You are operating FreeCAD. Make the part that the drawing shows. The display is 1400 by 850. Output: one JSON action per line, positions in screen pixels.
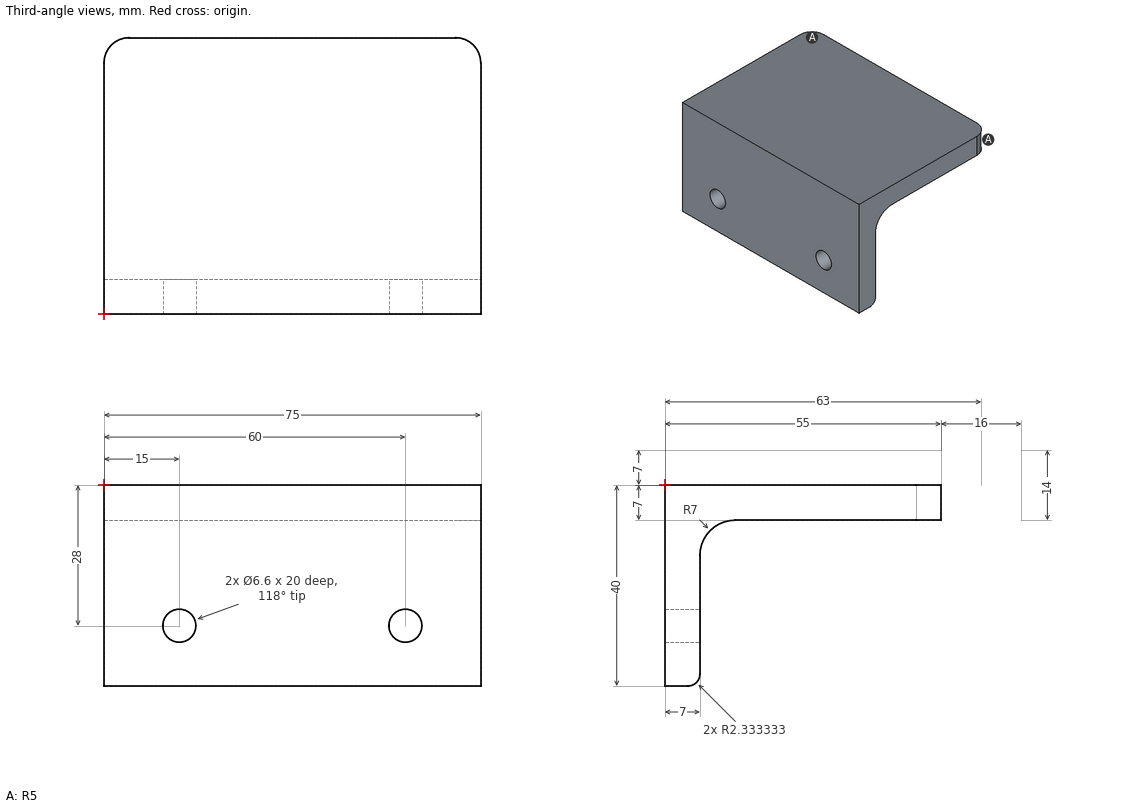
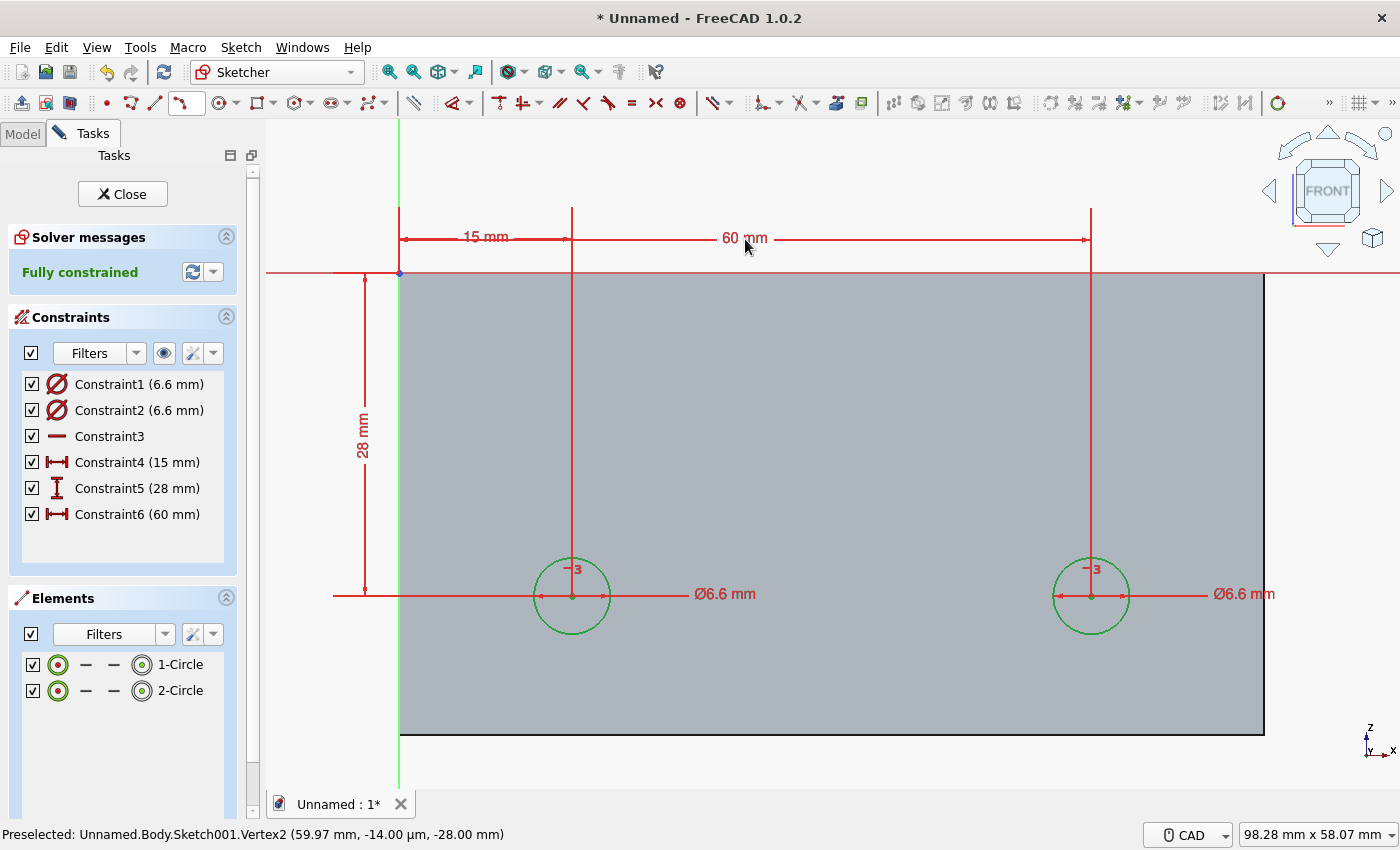
{"action": "left_click", "coordinate": [123, 194]}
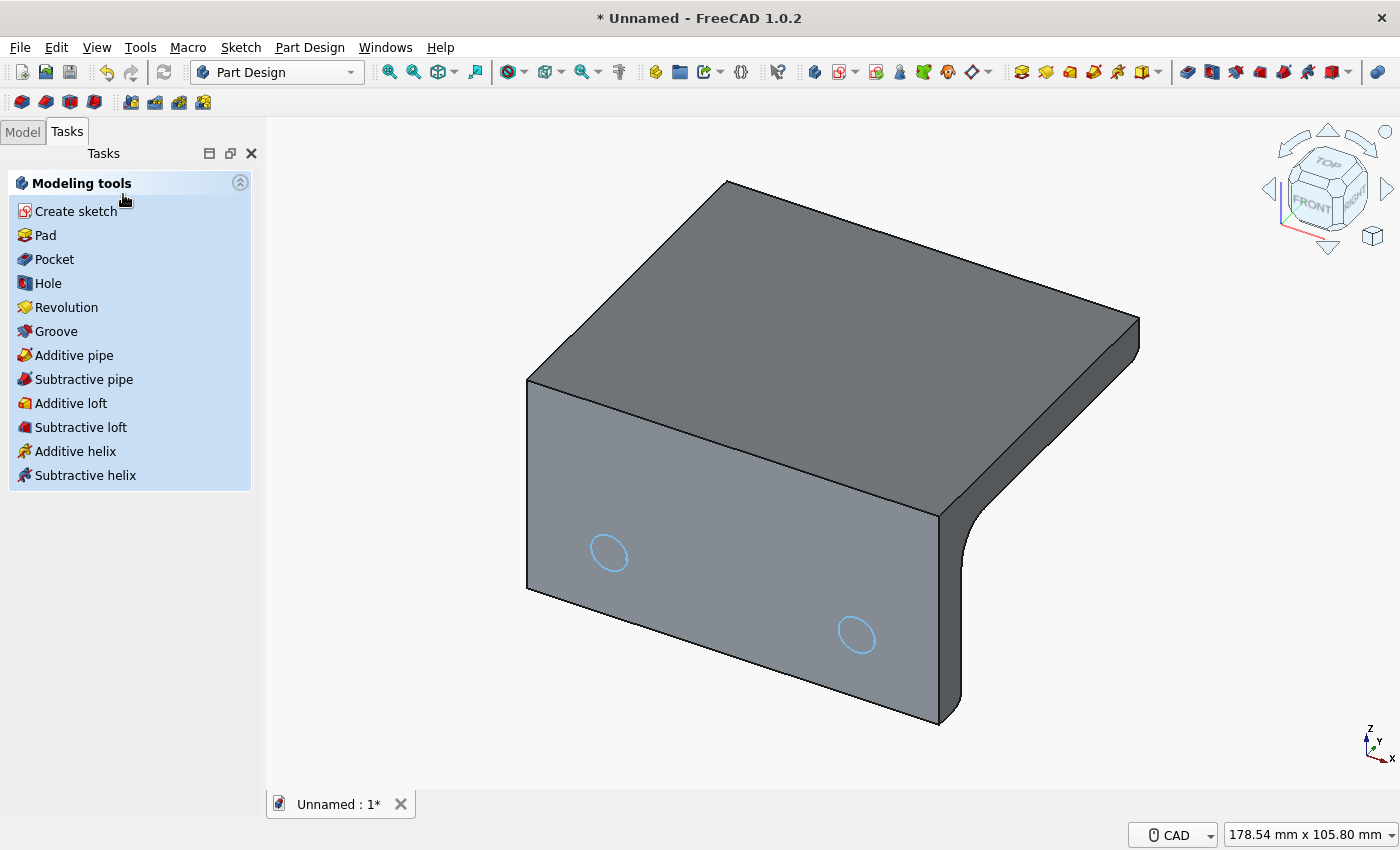
{"action": "left_click", "coordinate": [1212, 72]}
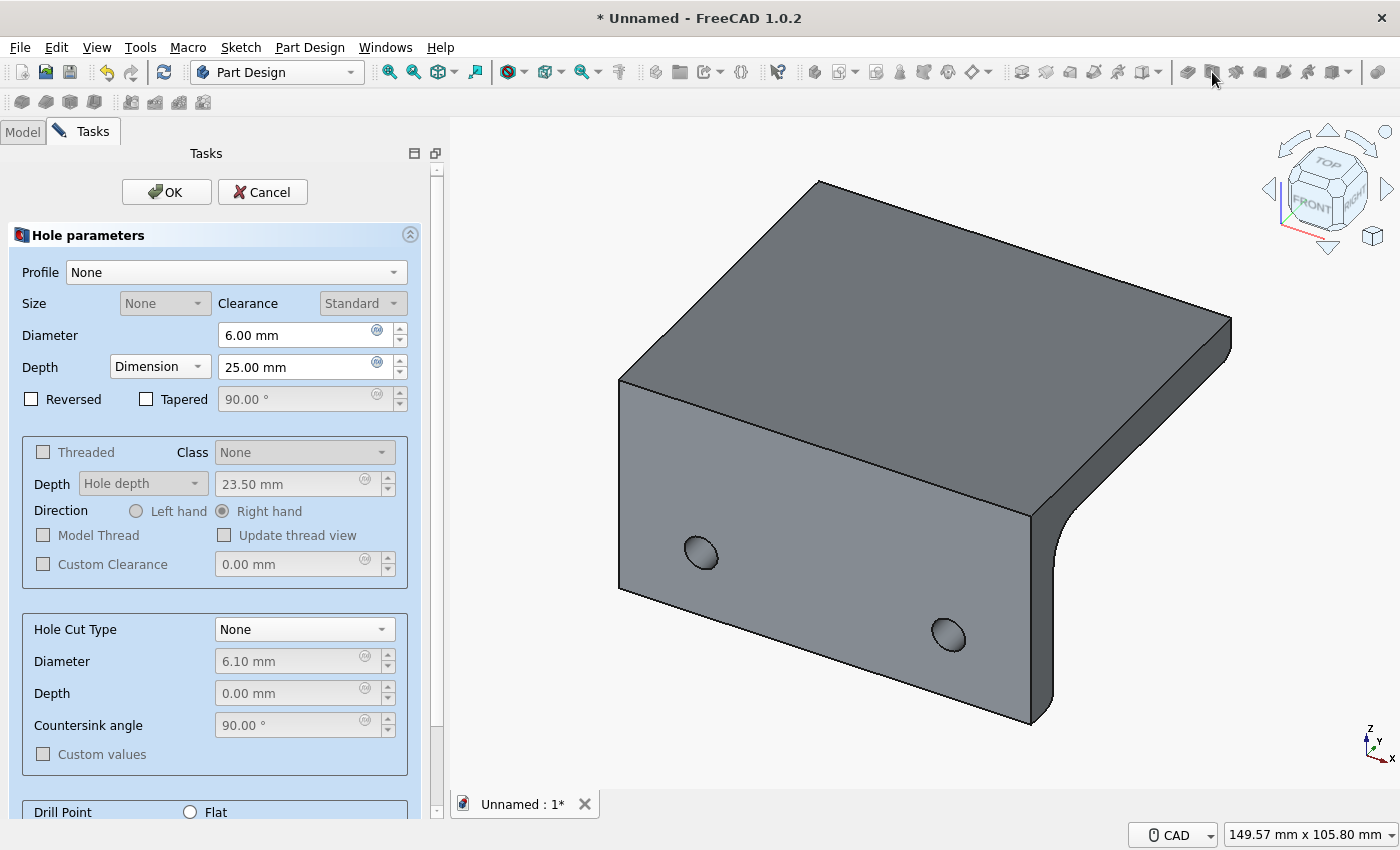
{"action": "triple_click", "coordinate": [305, 335]}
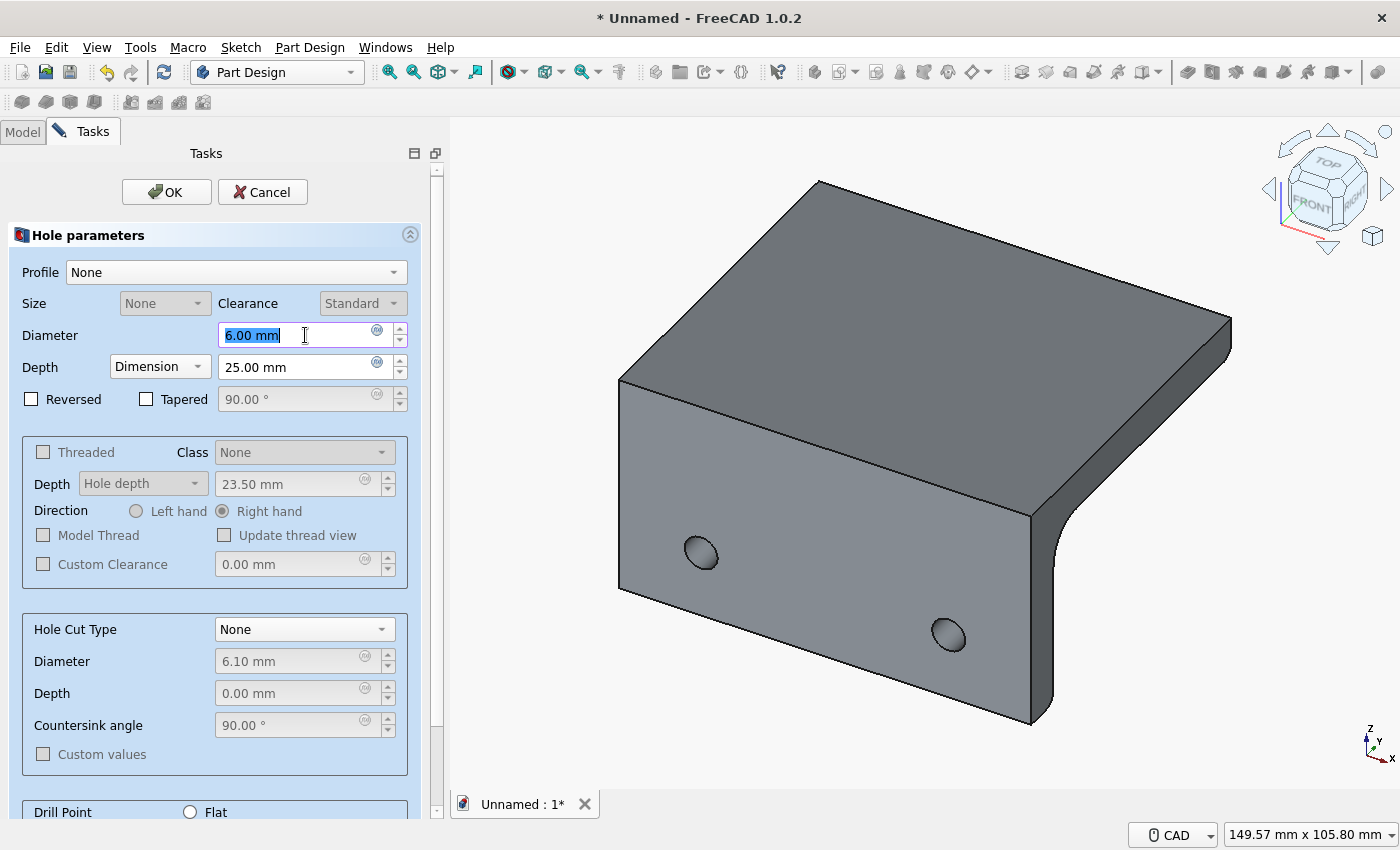
{"action": "type", "text": "6.6"}
{"action": "key", "text": "Tab"}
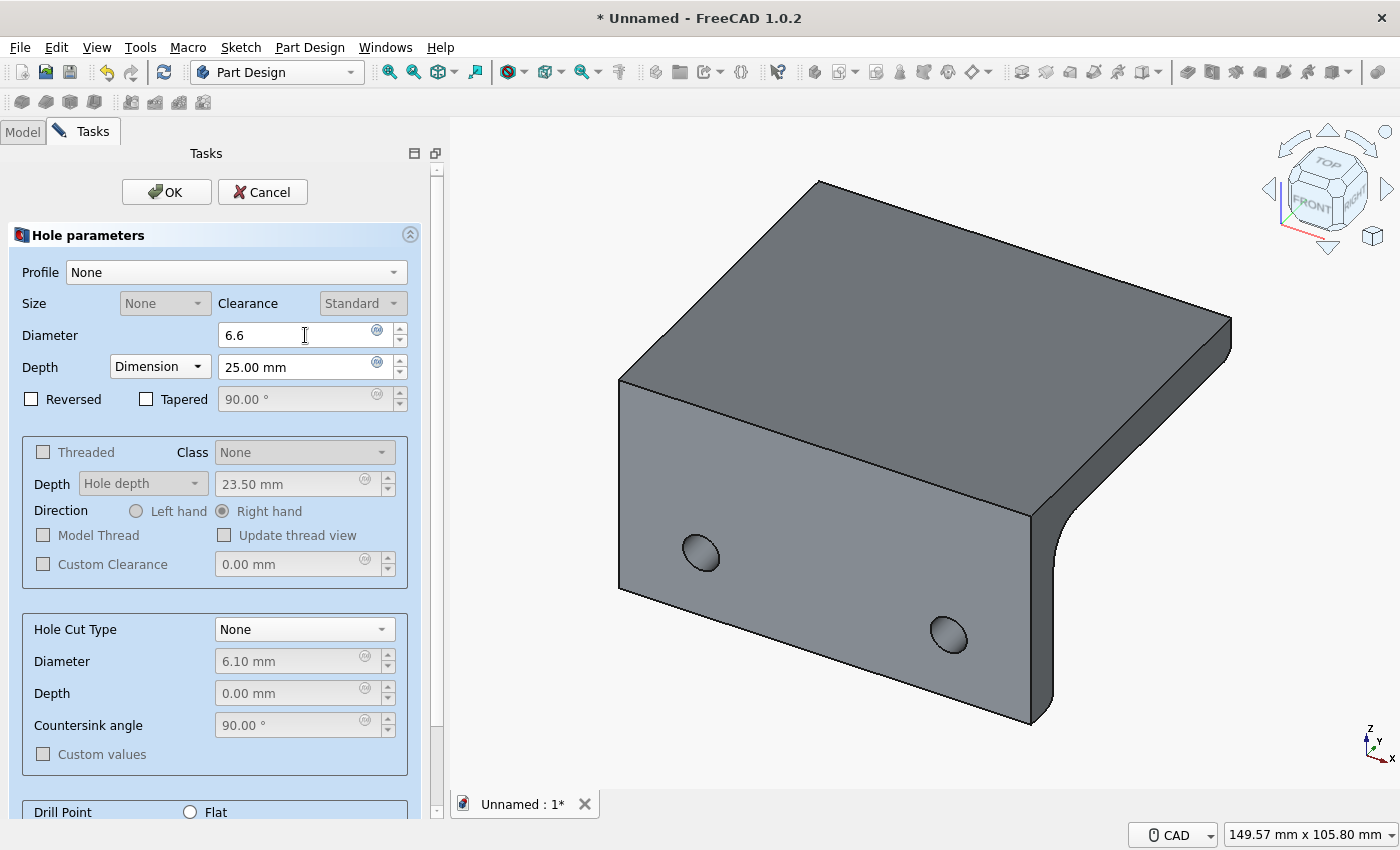
{"action": "triple_click", "coordinate": [305, 367]}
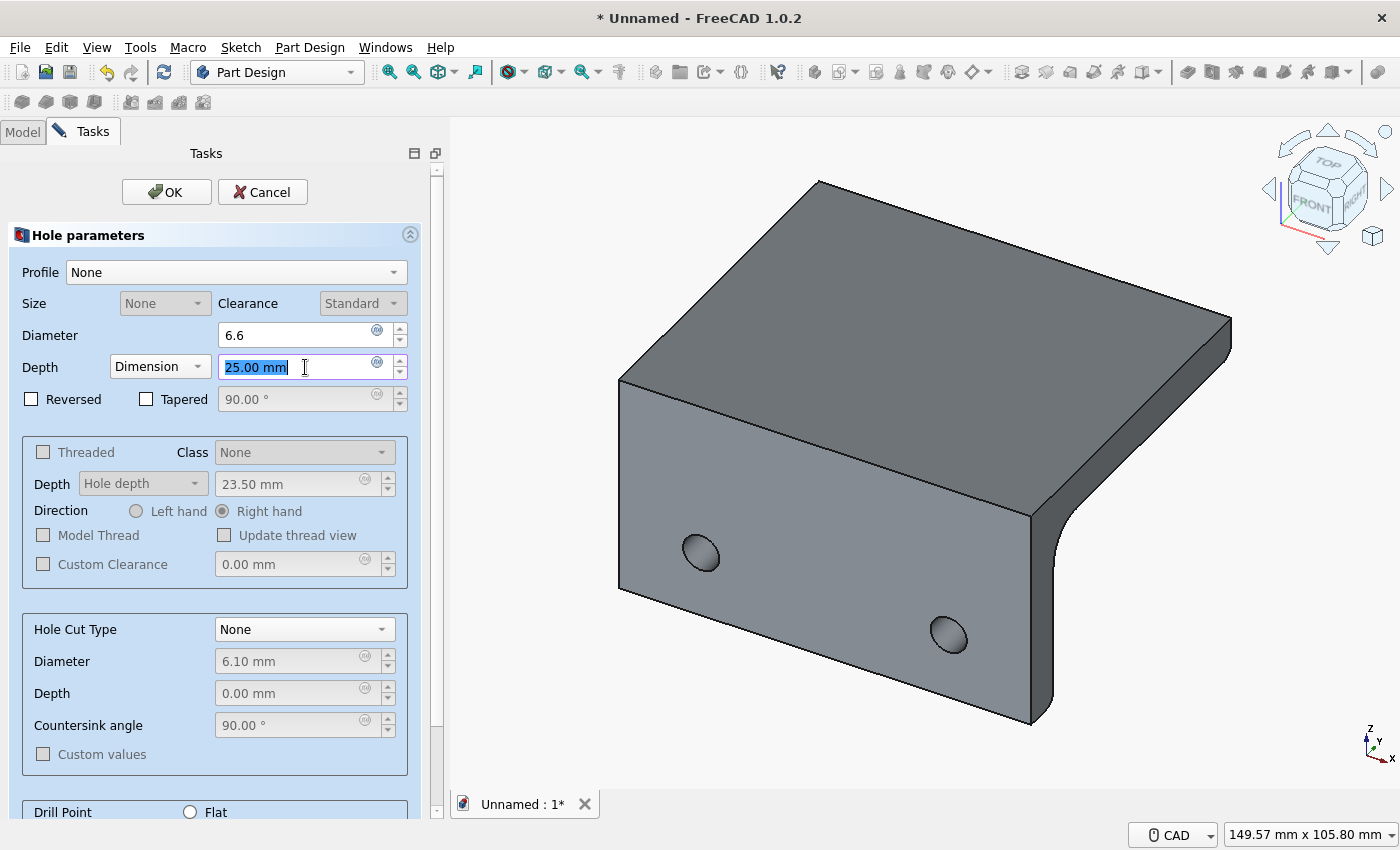
{"action": "type", "text": "20"}
{"action": "key", "text": "Tab"}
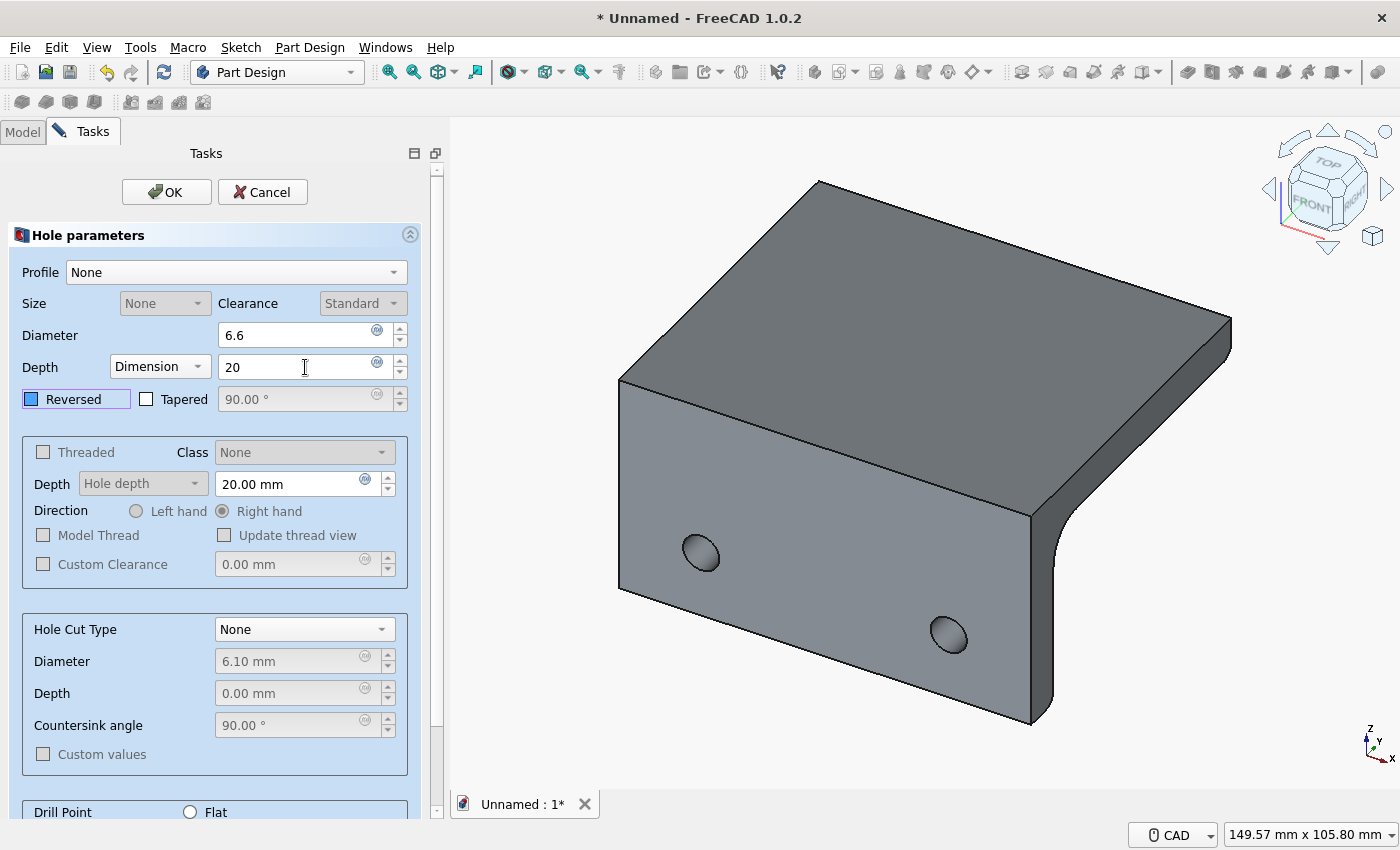
{"action": "left_click", "coordinate": [167, 192]}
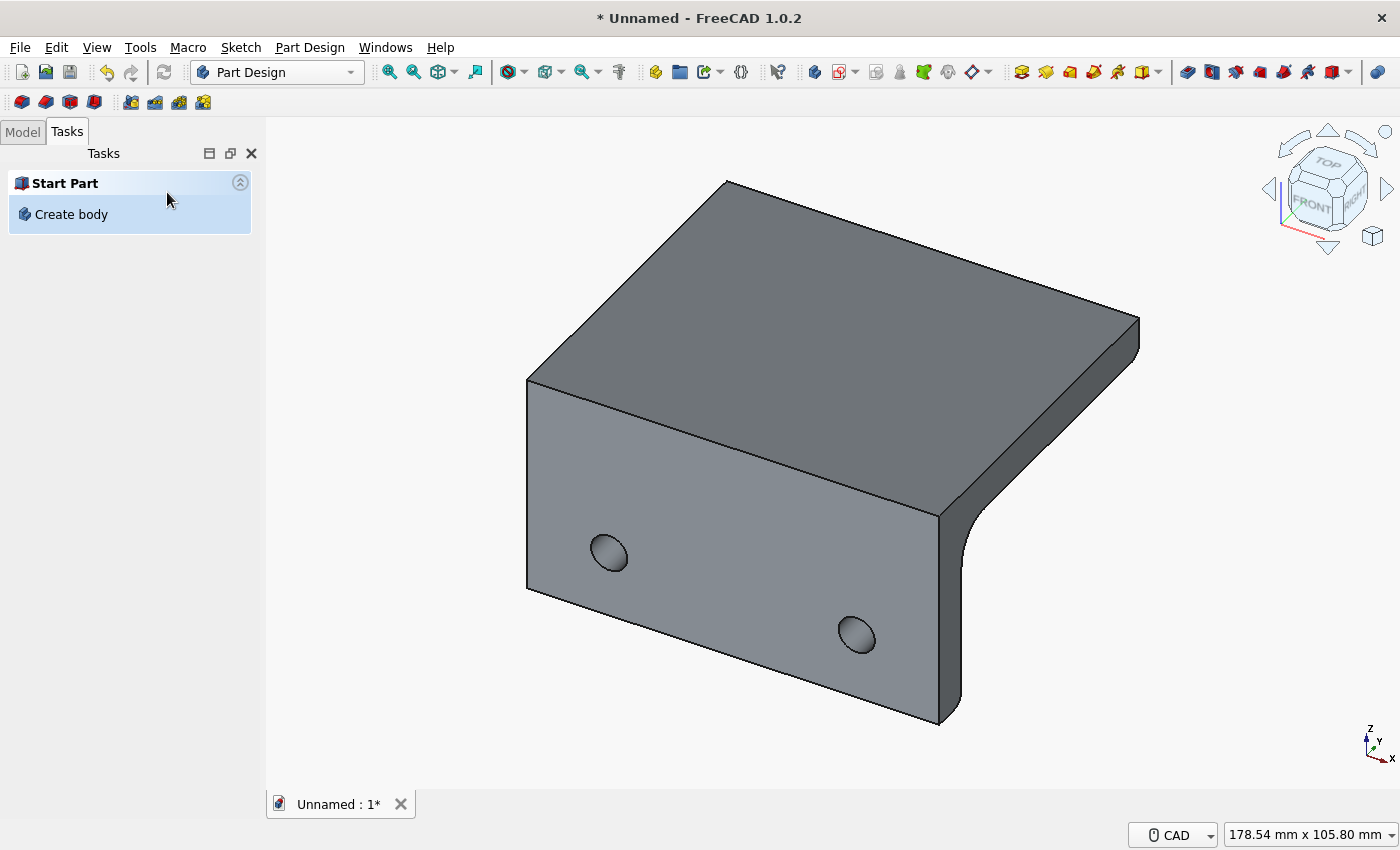
{"action": "left_click", "coordinate": [954, 546]}